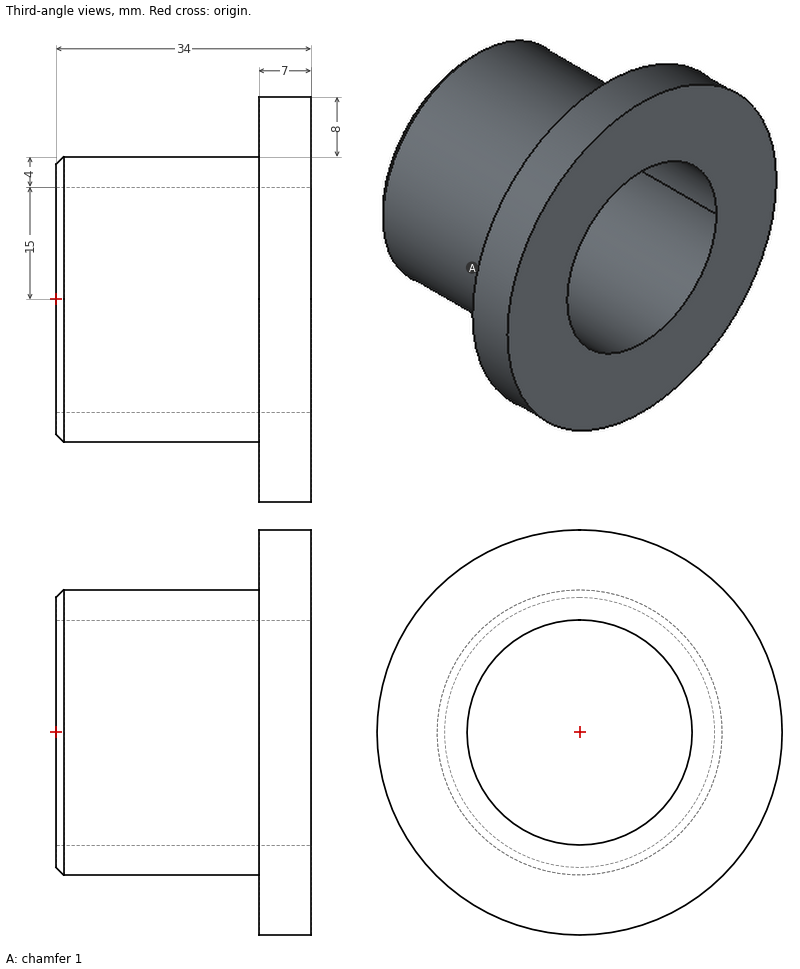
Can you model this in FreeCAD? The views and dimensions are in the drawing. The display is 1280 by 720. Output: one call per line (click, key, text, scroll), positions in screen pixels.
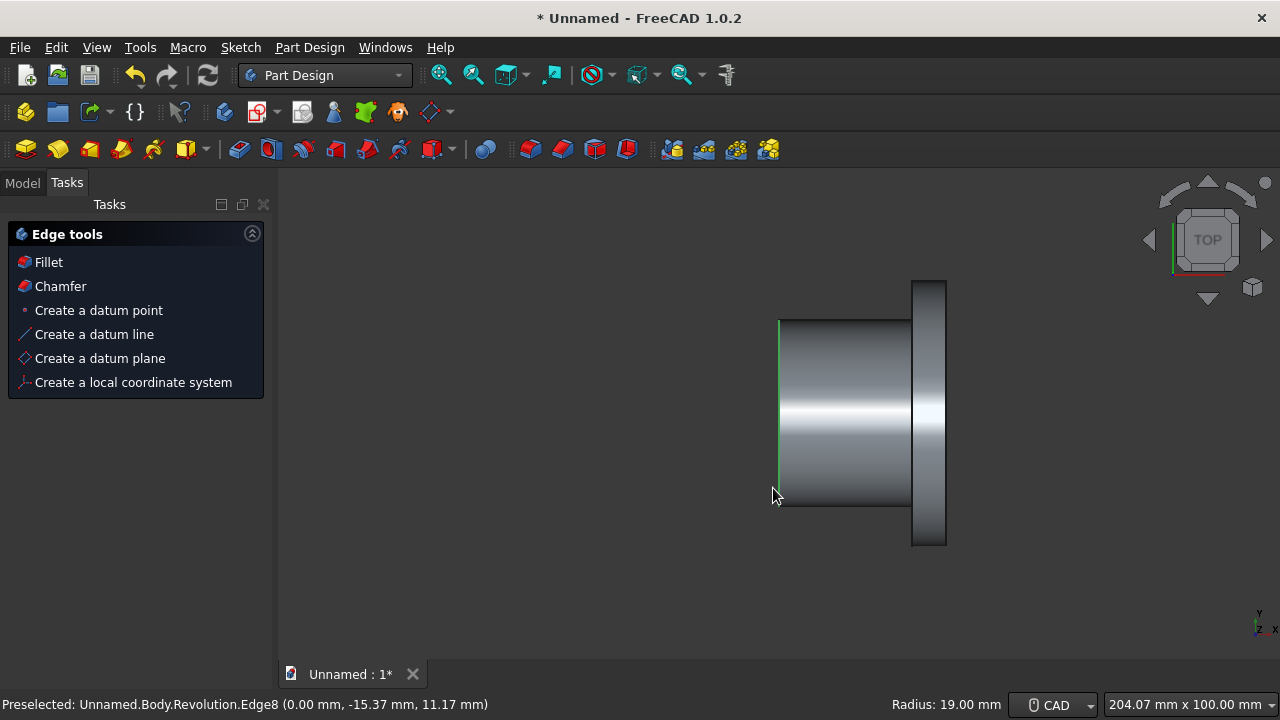
click(564, 150)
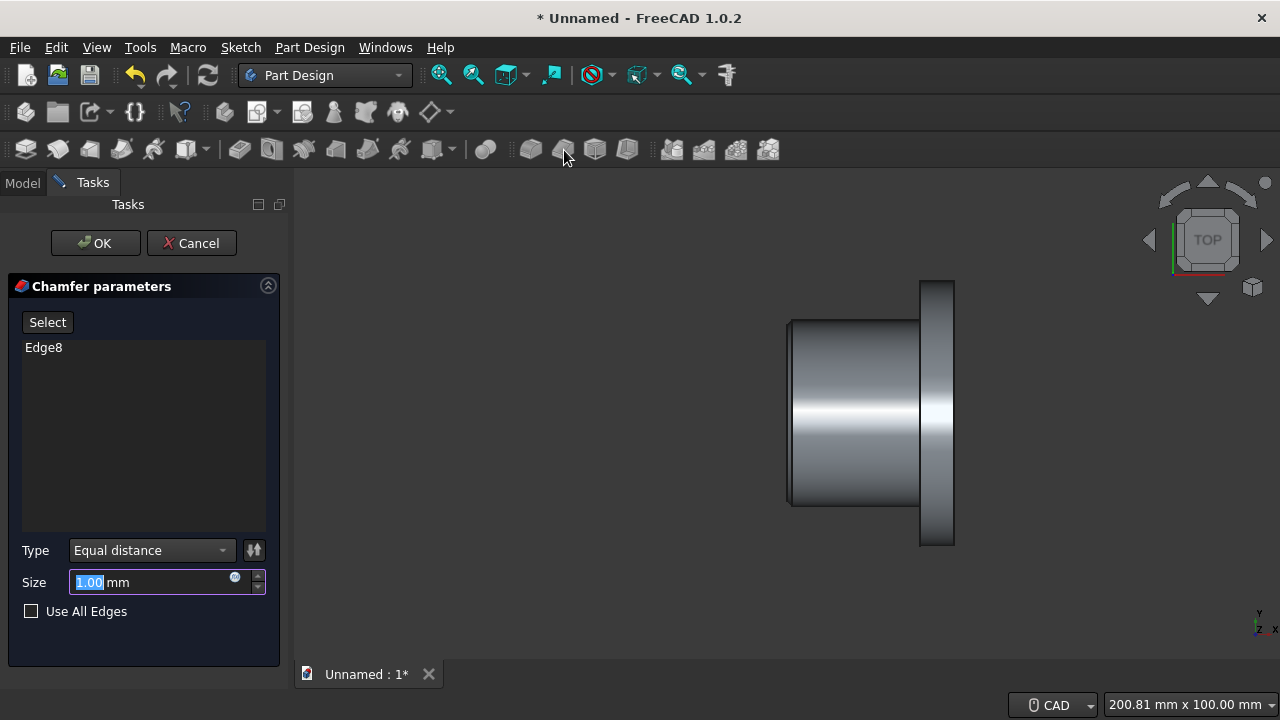
text(1)
key(Tab)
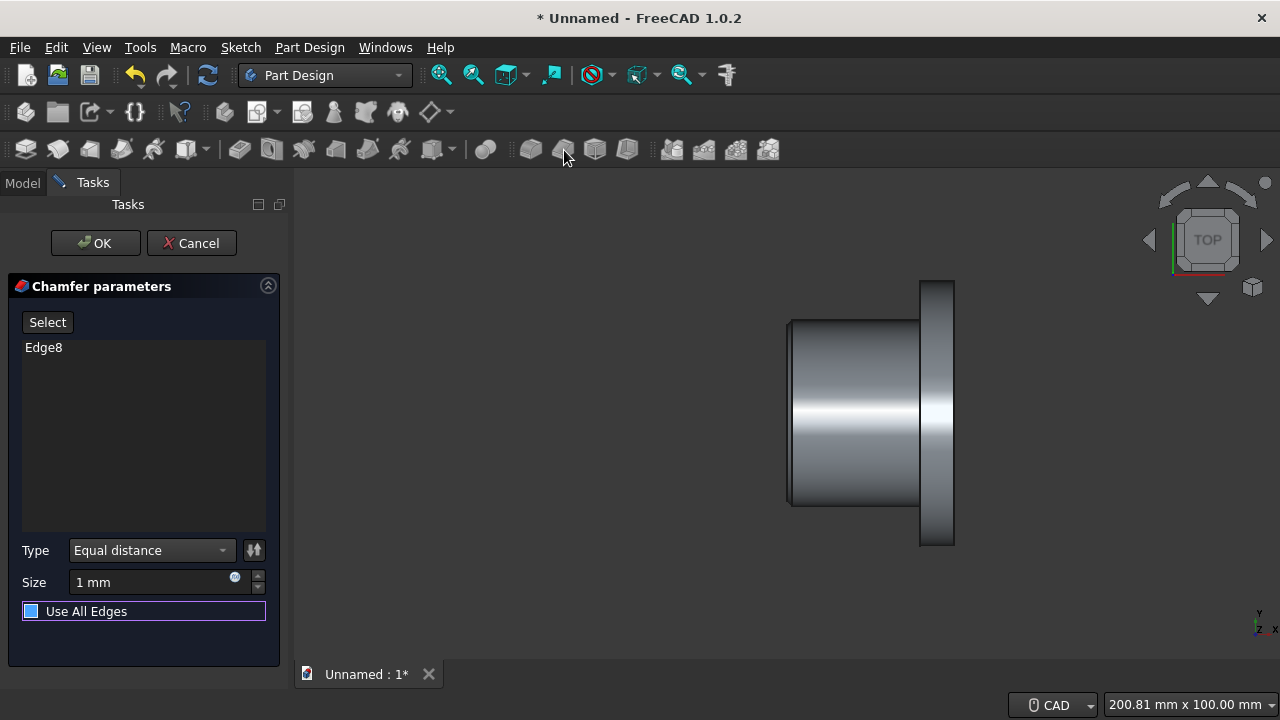
click(96, 243)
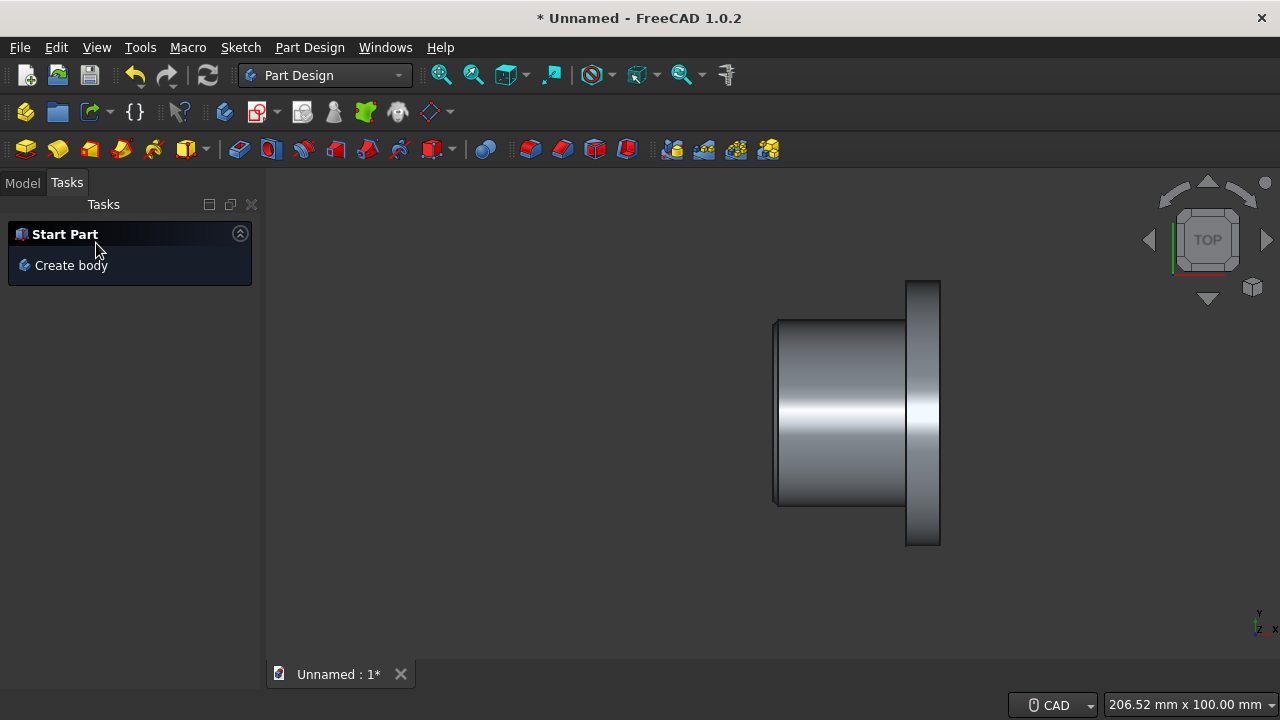
key(0)